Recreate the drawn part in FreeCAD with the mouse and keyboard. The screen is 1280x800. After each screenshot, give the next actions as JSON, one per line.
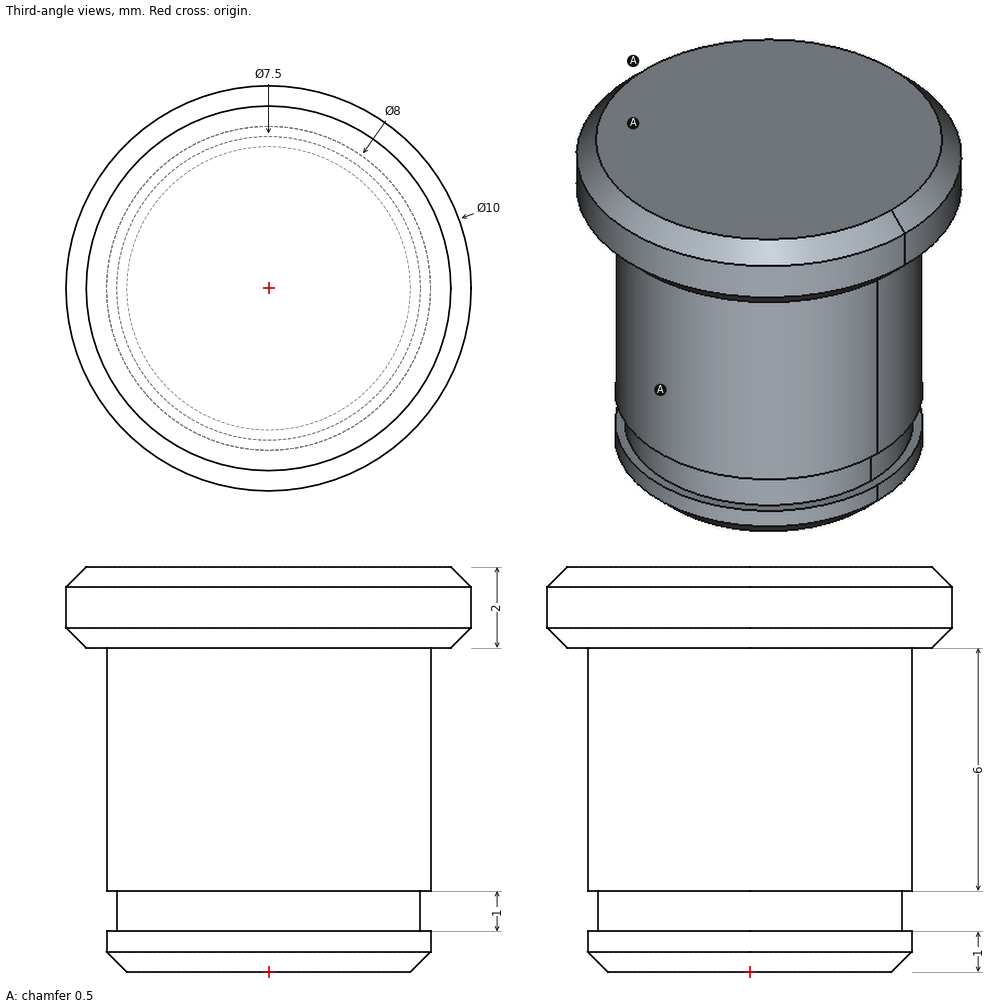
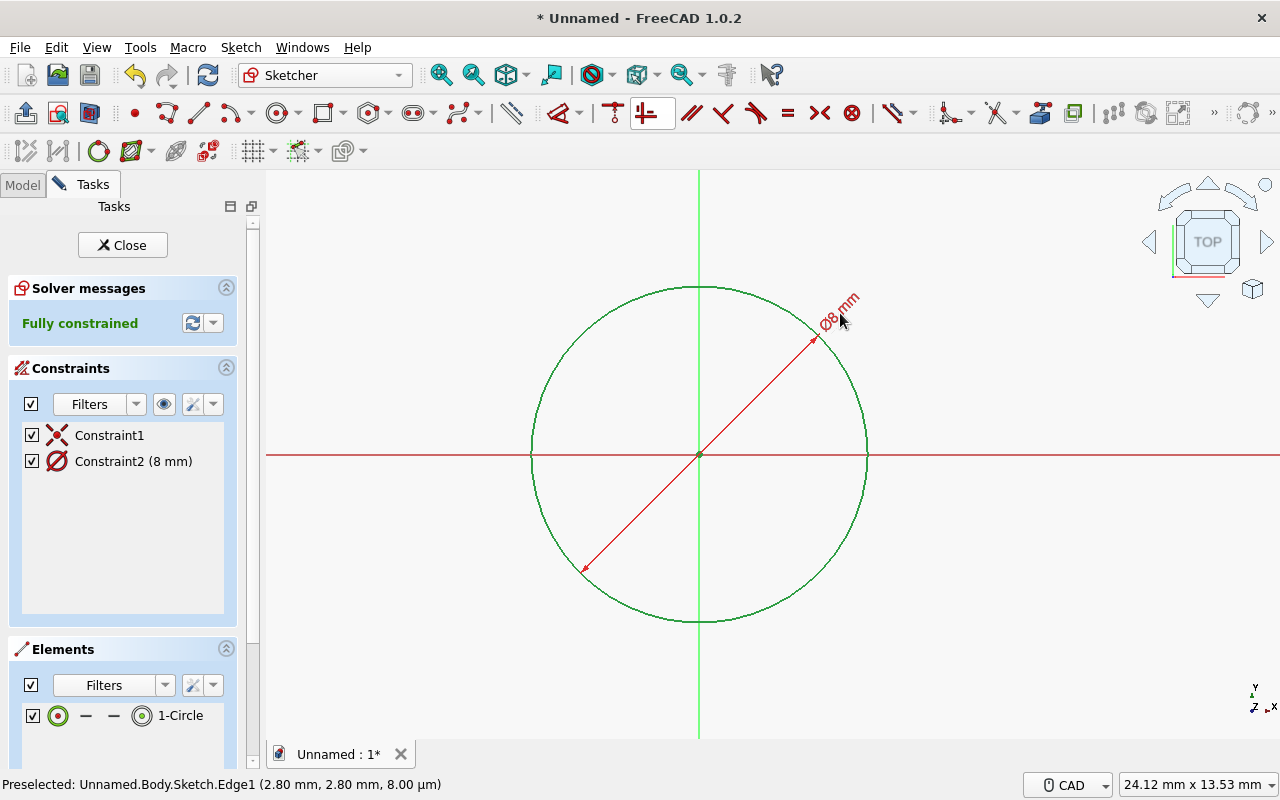
{"action": "left_click", "coordinate": [123, 245]}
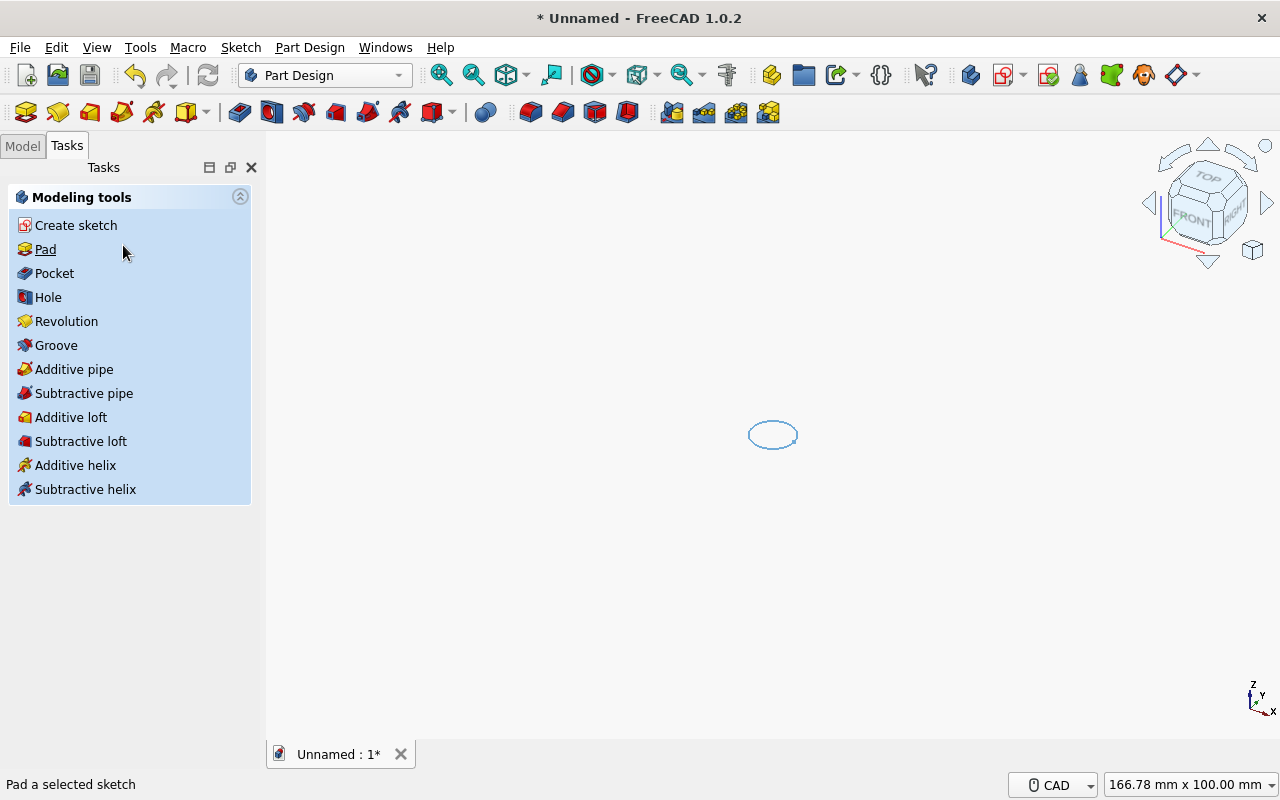
{"action": "left_click", "coordinate": [26, 112]}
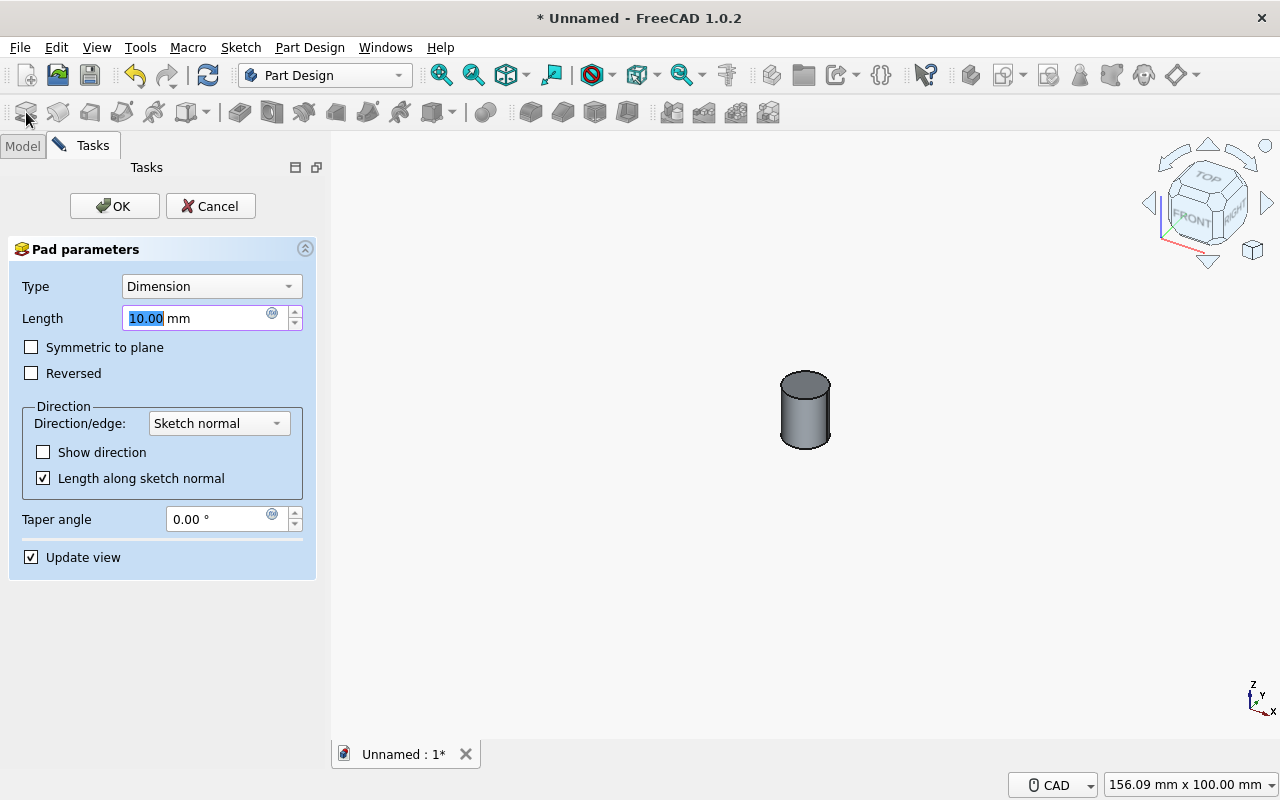
{"action": "type", "text": "1"}
{"action": "key", "text": "Tab"}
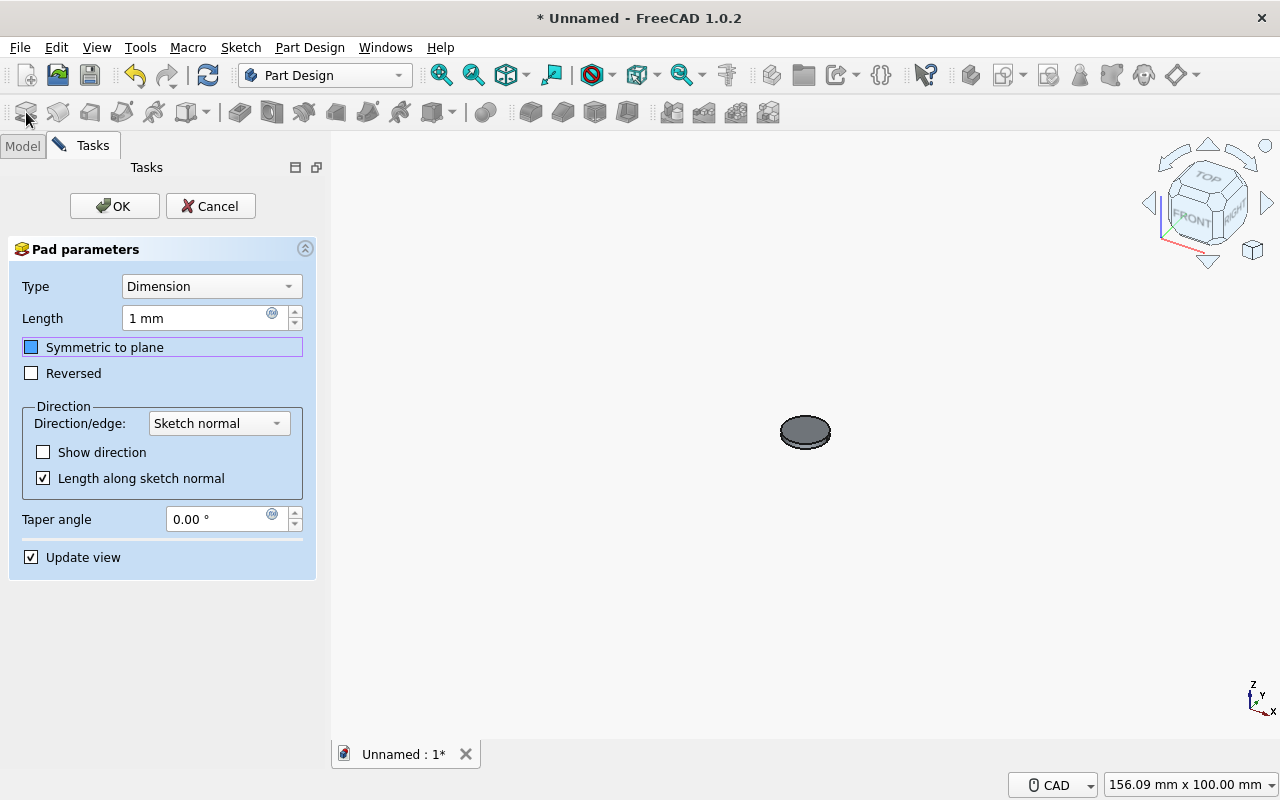
{"action": "left_click", "coordinate": [115, 206]}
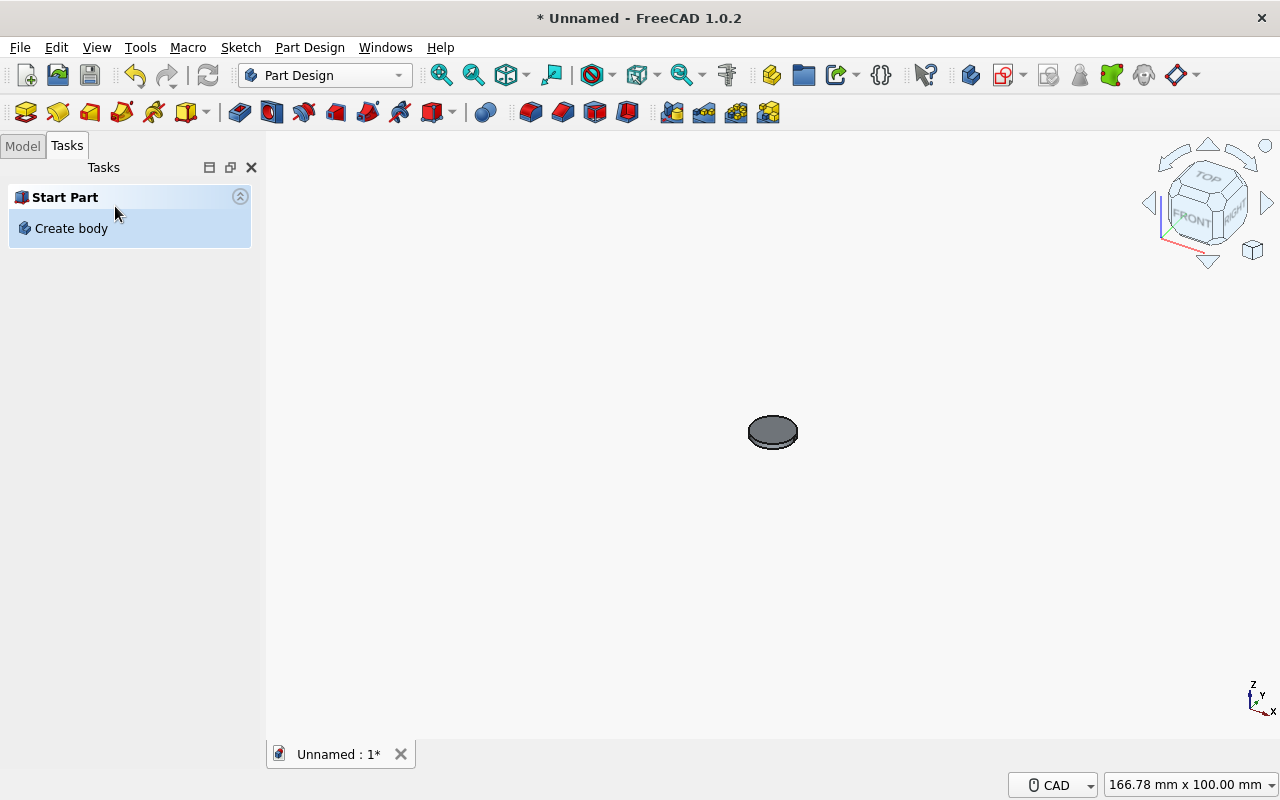
{"action": "key", "text": "v f"}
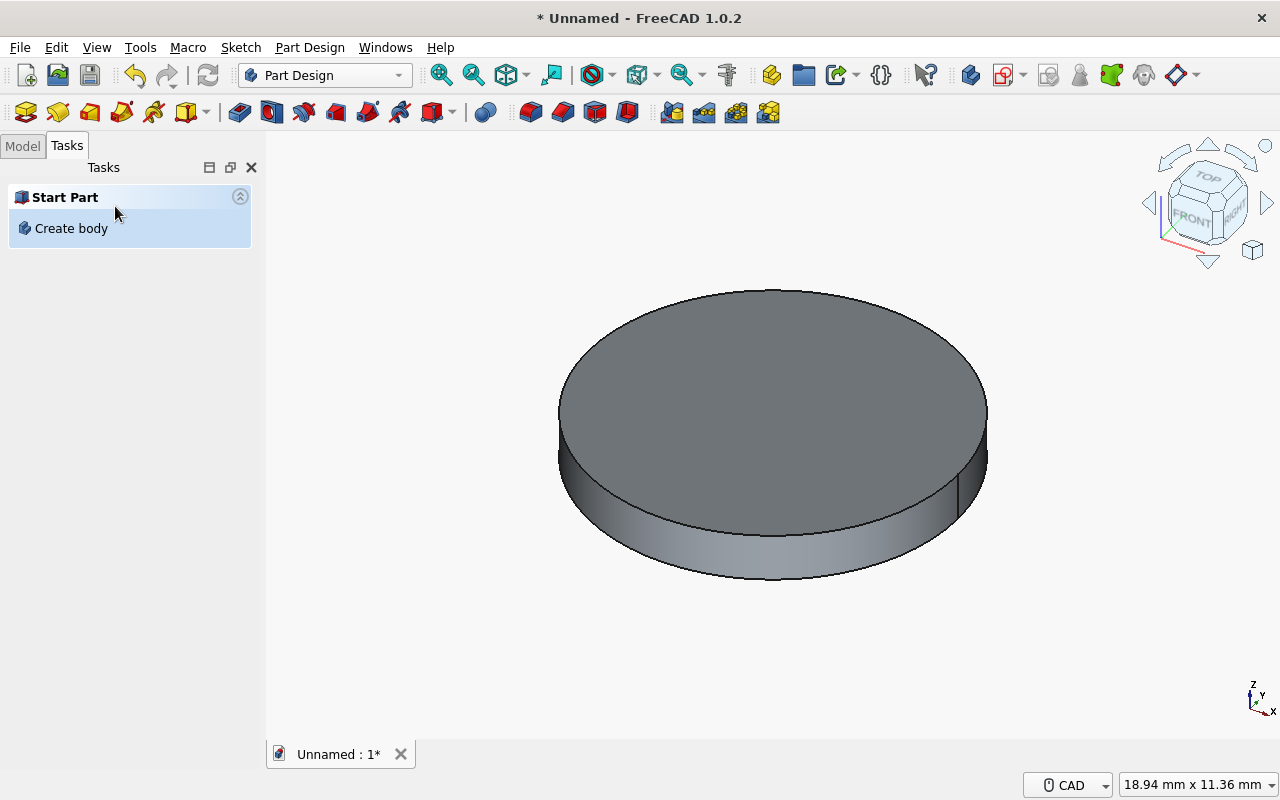
{"action": "left_click", "coordinate": [773, 412]}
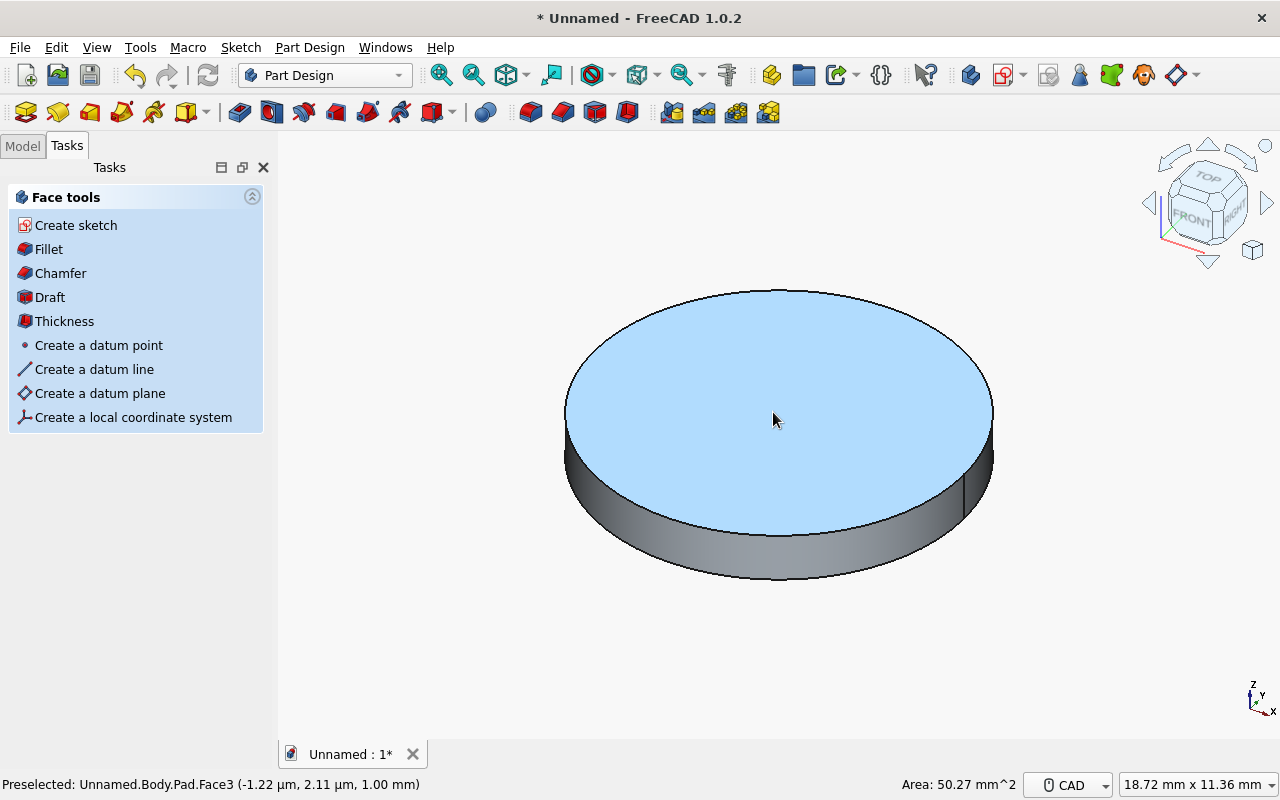
{"action": "left_click", "coordinate": [1004, 76]}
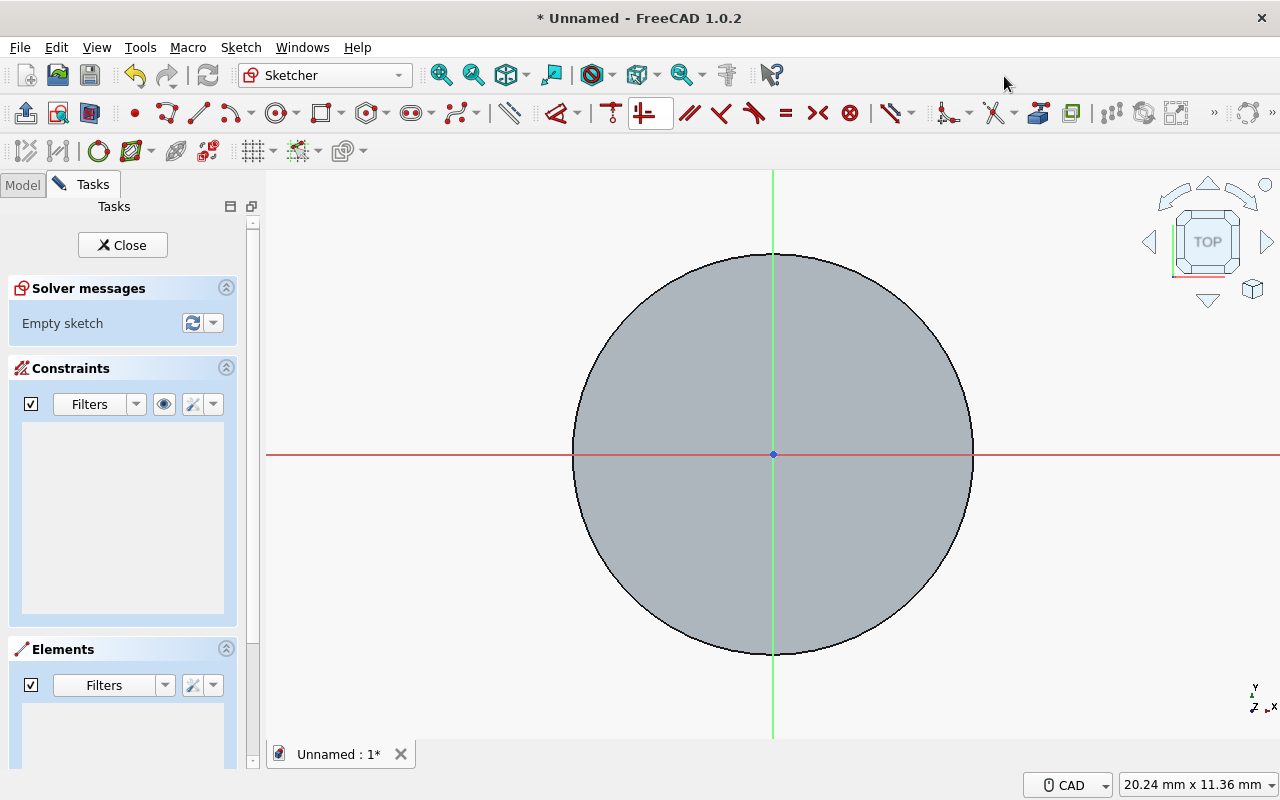
{"action": "key", "text": "g c"}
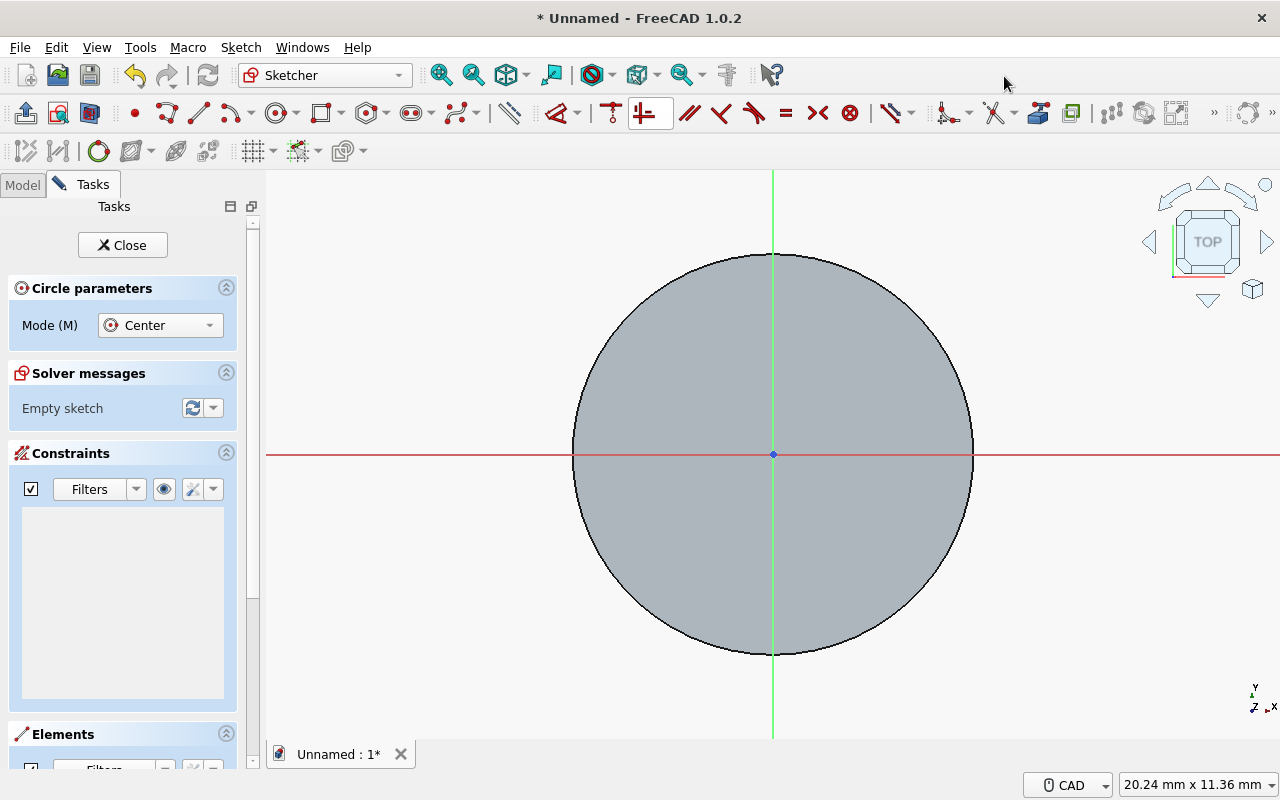
{"action": "left_click", "coordinate": [773, 454]}
{"action": "left_click", "coordinate": [906, 322]}
{"action": "key", "text": "Escape"}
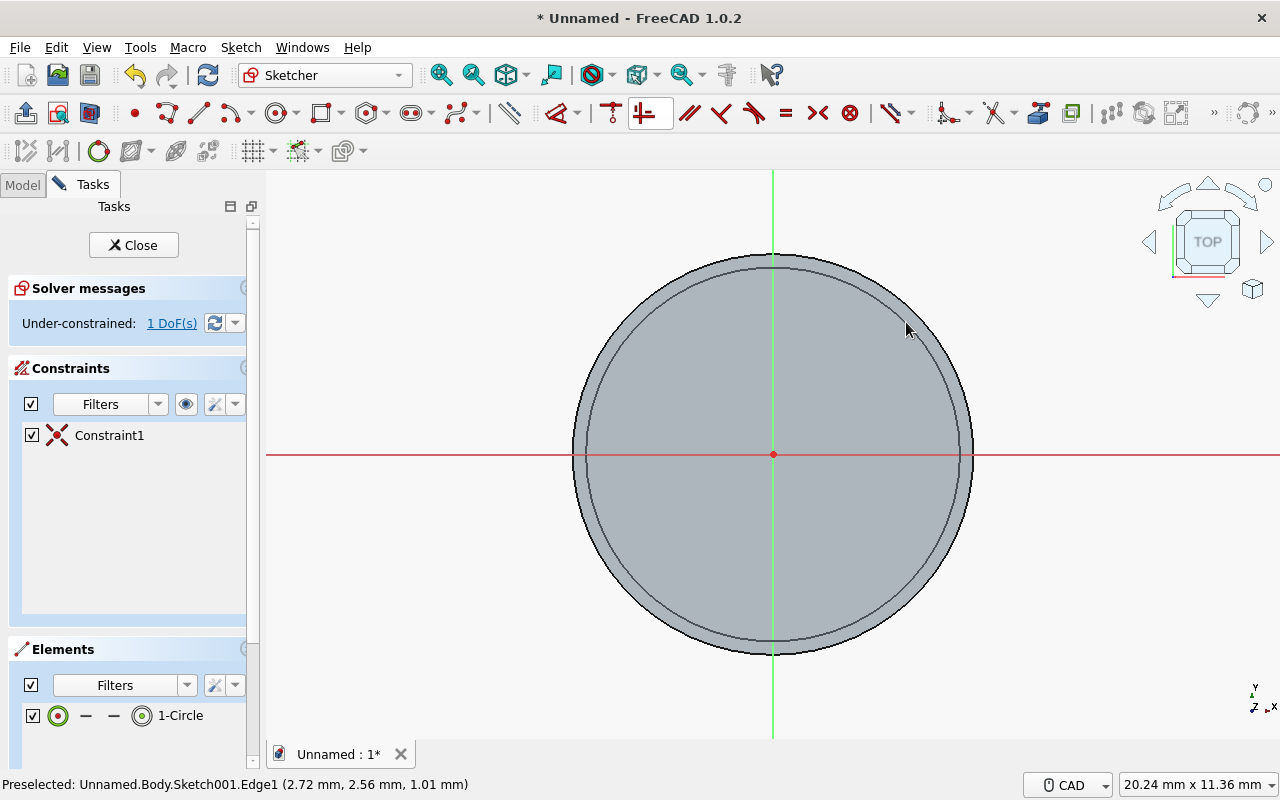
{"action": "key", "text": "d"}